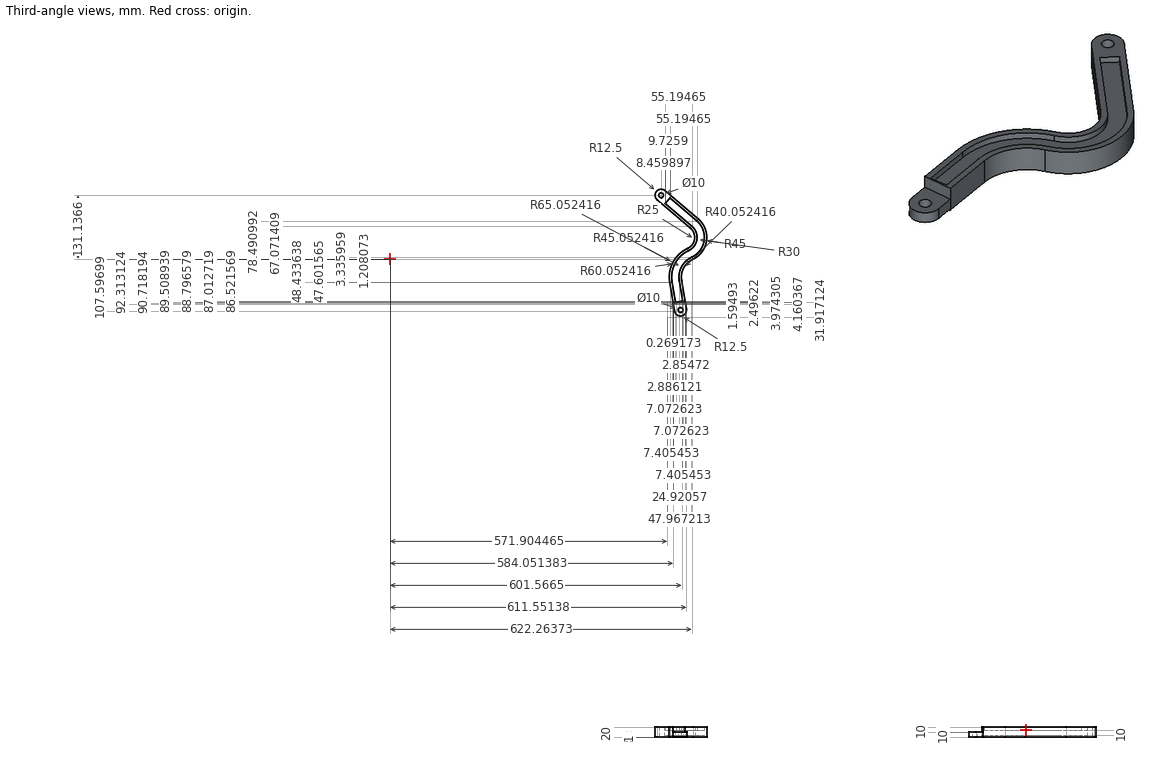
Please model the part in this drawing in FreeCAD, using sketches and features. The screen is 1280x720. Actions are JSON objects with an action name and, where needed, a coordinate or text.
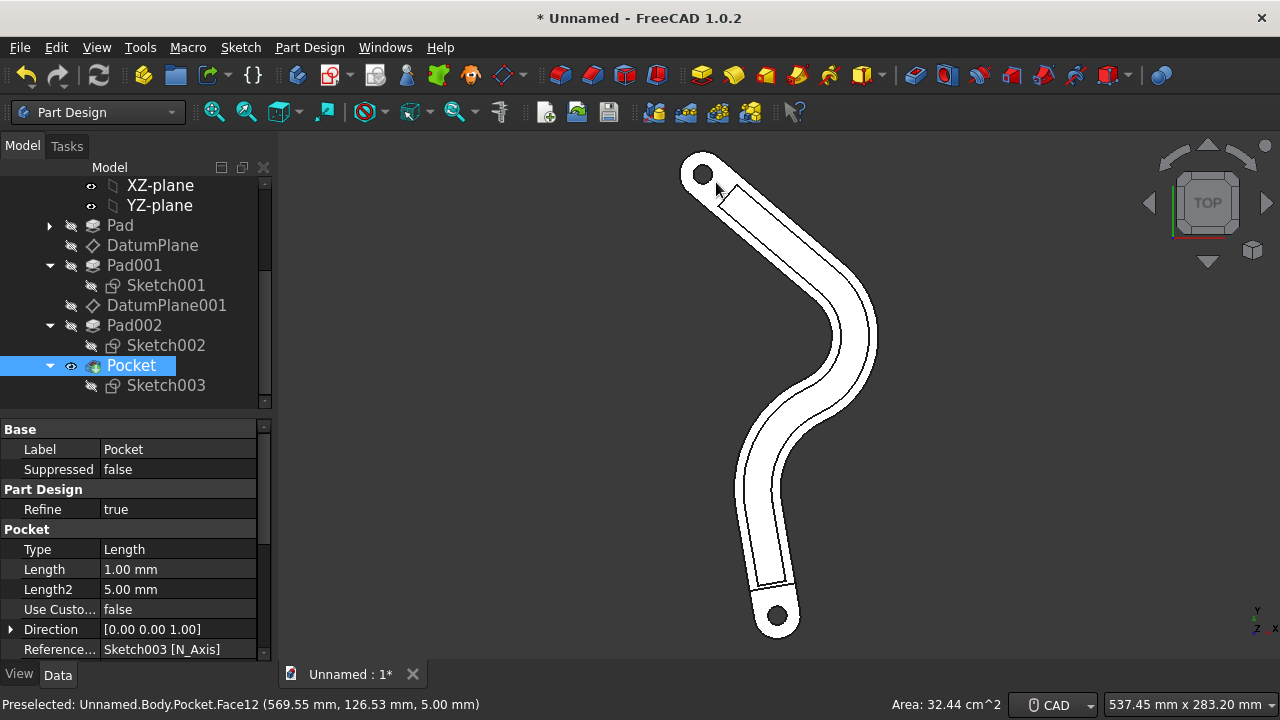
{"action": "left_click", "coordinate": [330, 76]}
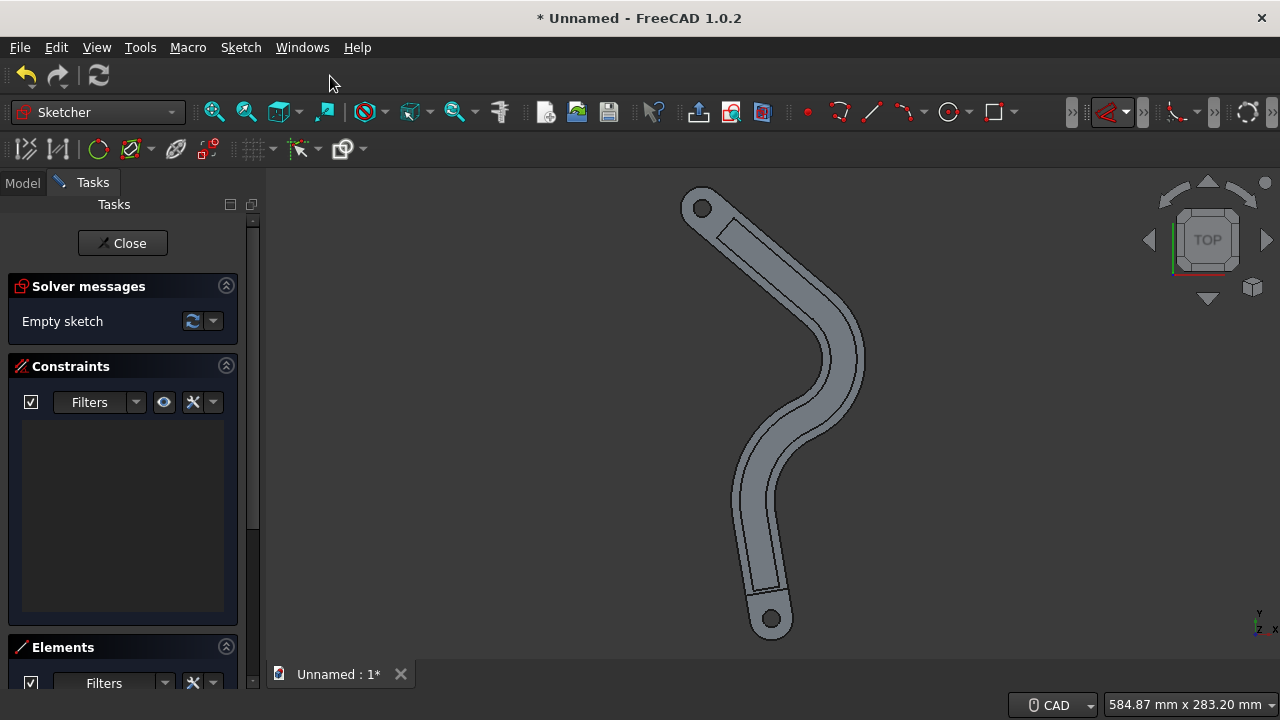
{"action": "scroll", "coordinate": [772, 606], "scroll_direction": "up", "scroll_amount": 13}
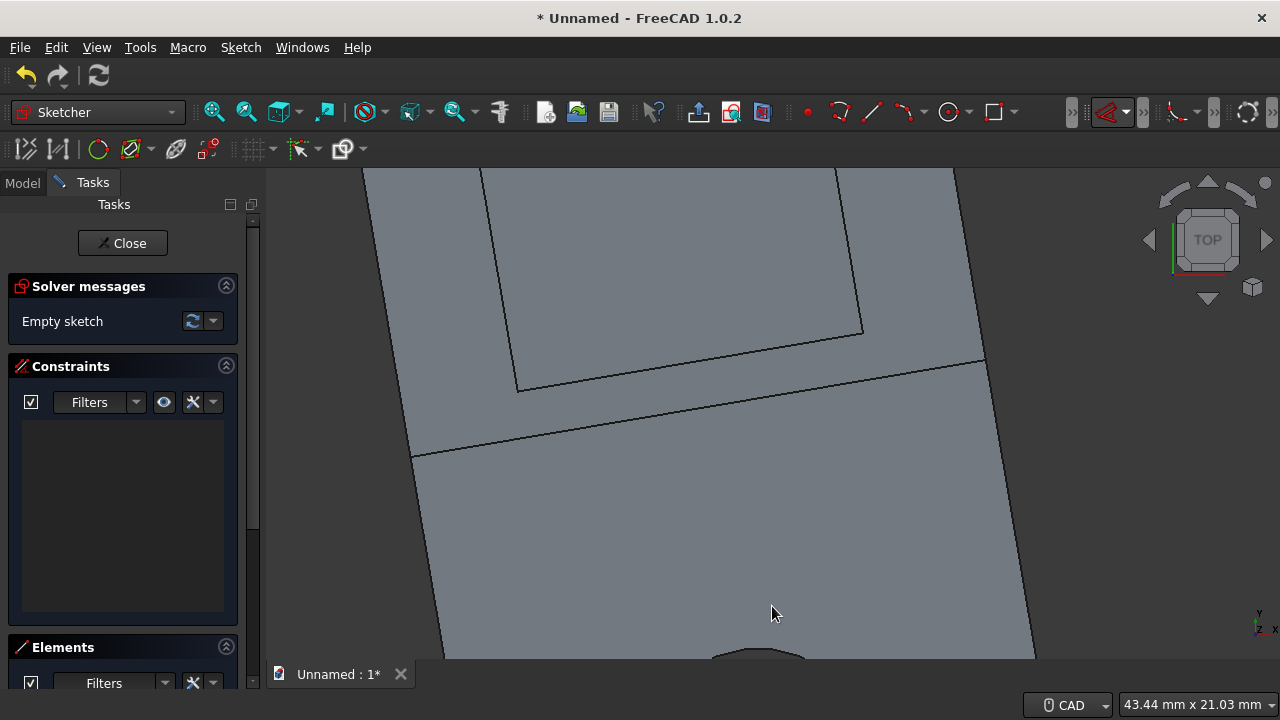
{"action": "left_click", "coordinate": [840, 112]}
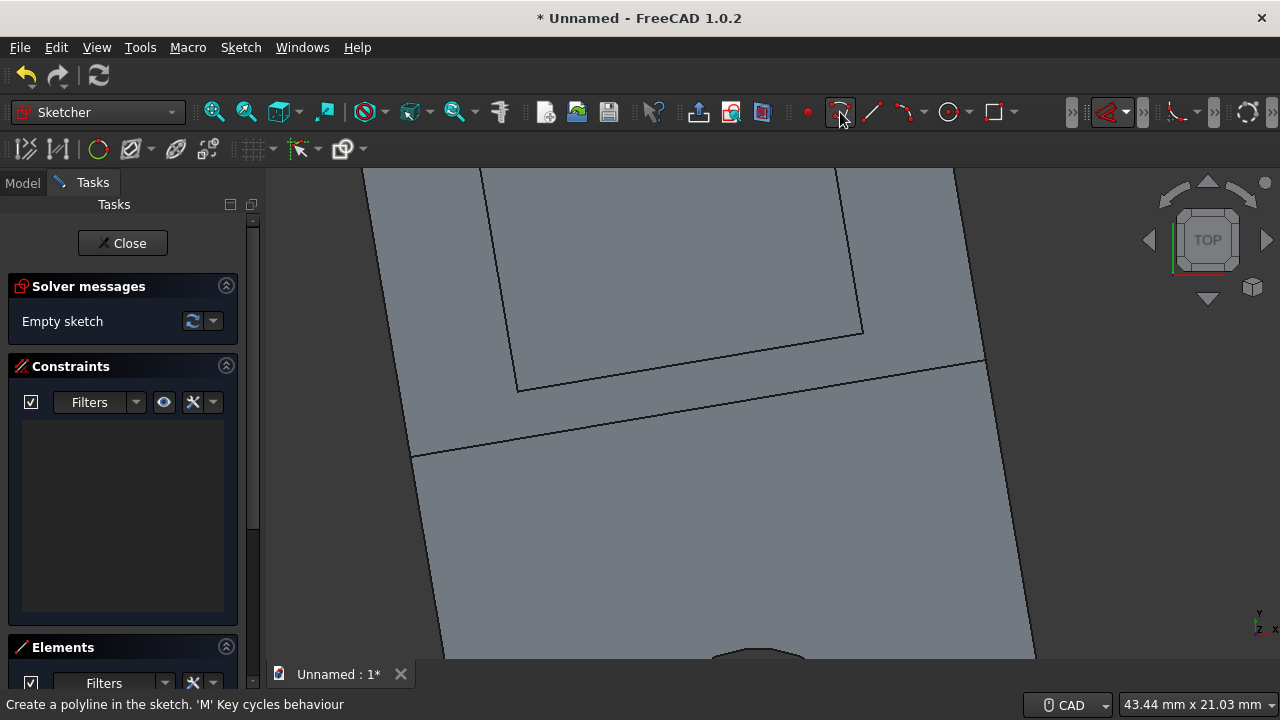
{"action": "left_click", "coordinate": [404, 420]}
{"action": "left_click", "coordinate": [410, 457]}
{"action": "left_click", "coordinate": [986, 360]}
{"action": "left_click", "coordinate": [404, 421]}
{"action": "key", "text": "Escape"}
{"action": "key", "text": "Escape"}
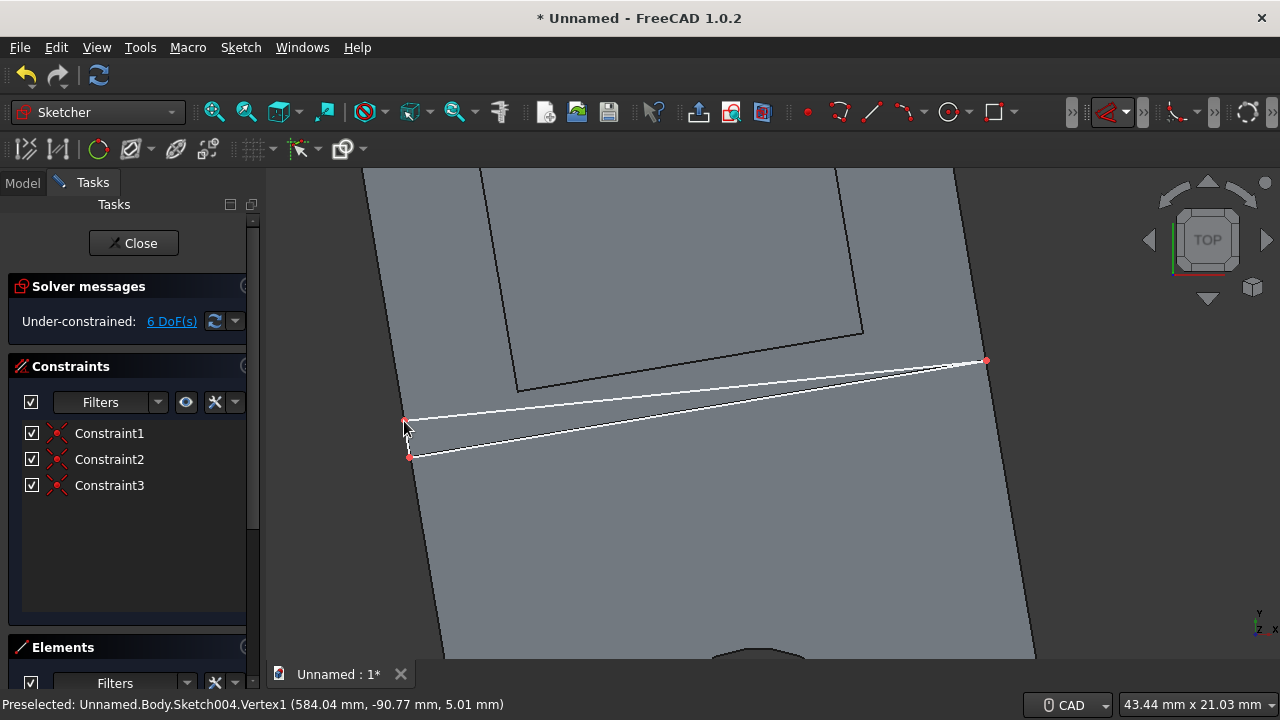
{"action": "scroll", "coordinate": [406, 432], "scroll_direction": "up", "scroll_amount": 2}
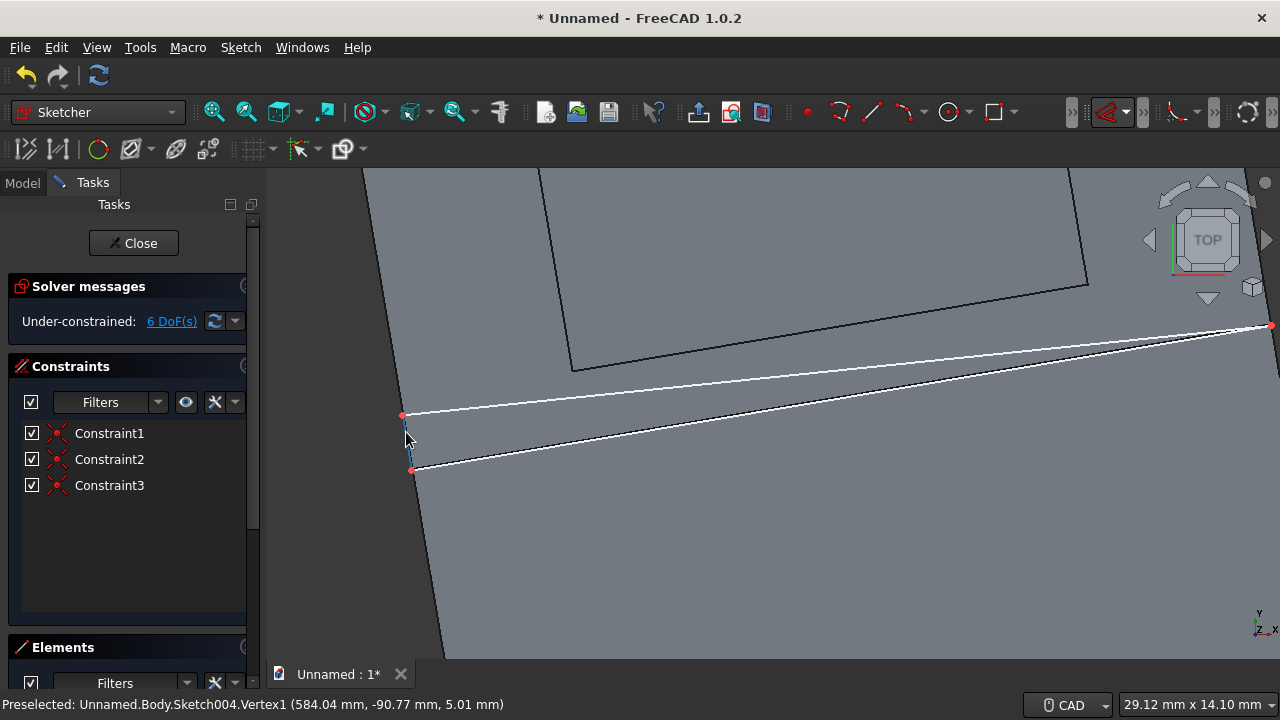
{"action": "left_click", "coordinate": [406, 432]}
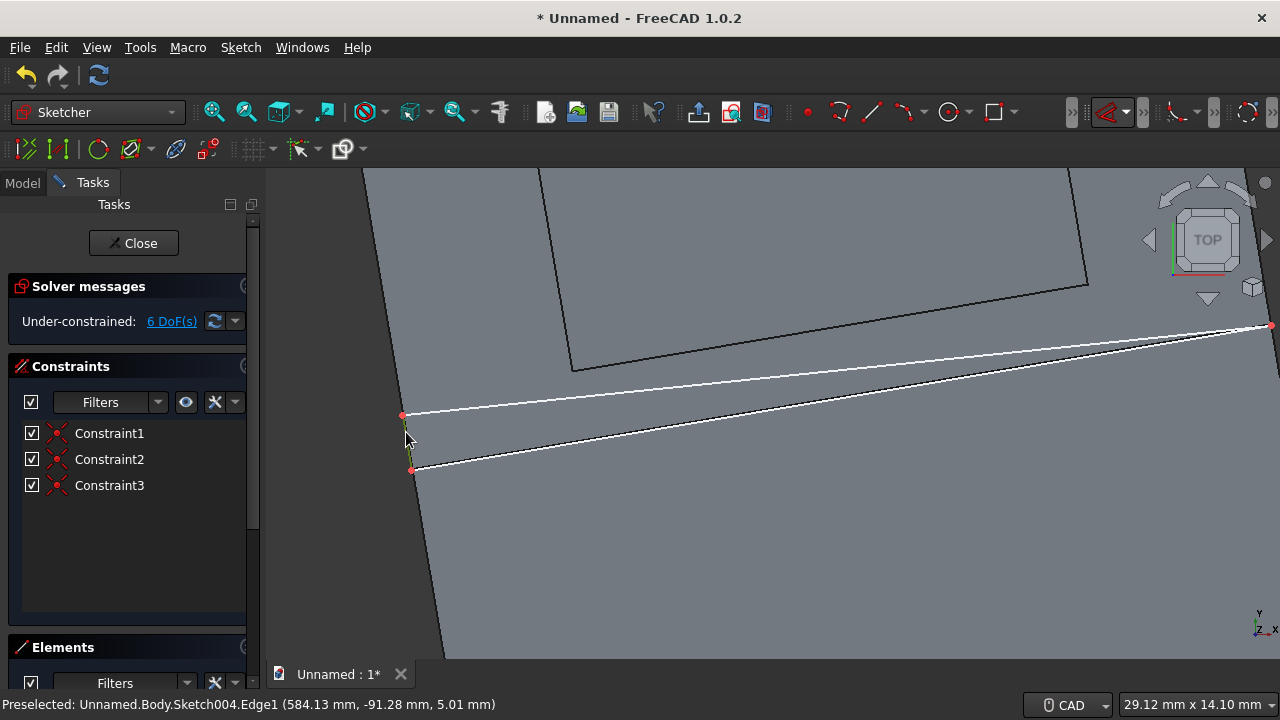
{"action": "left_click", "coordinate": [1128, 112]}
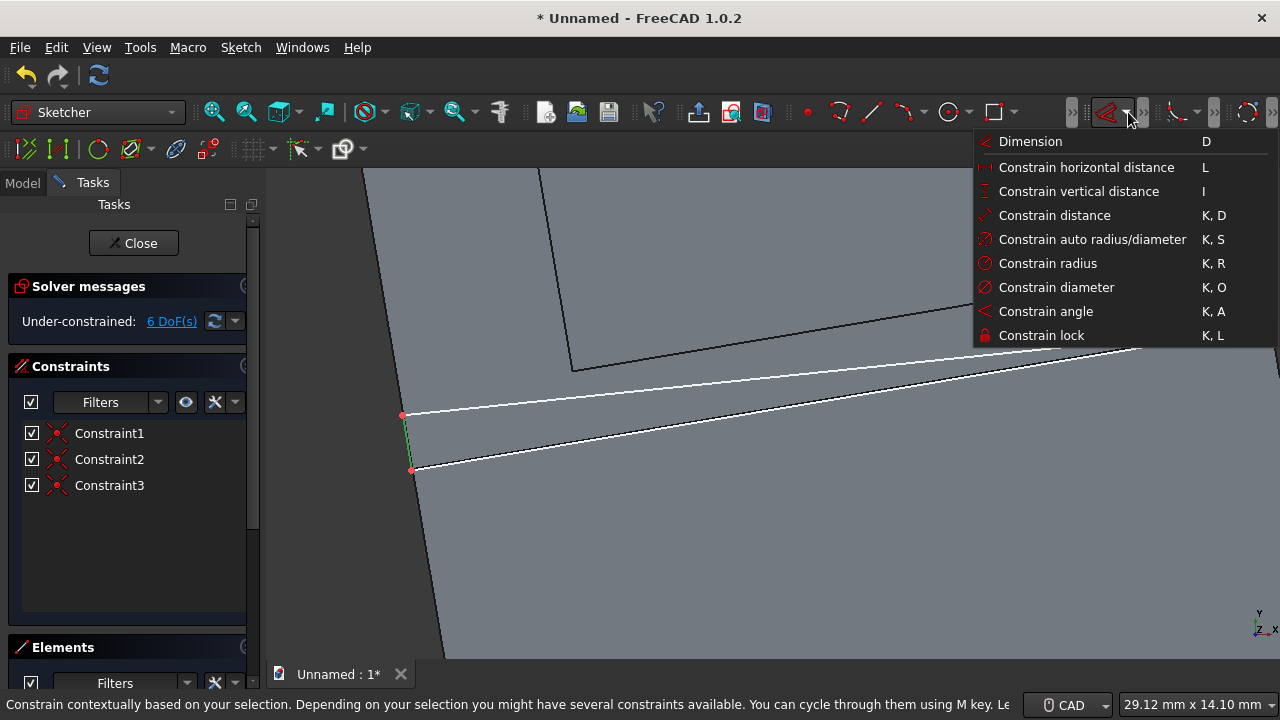
{"action": "left_click", "coordinate": [1126, 191]}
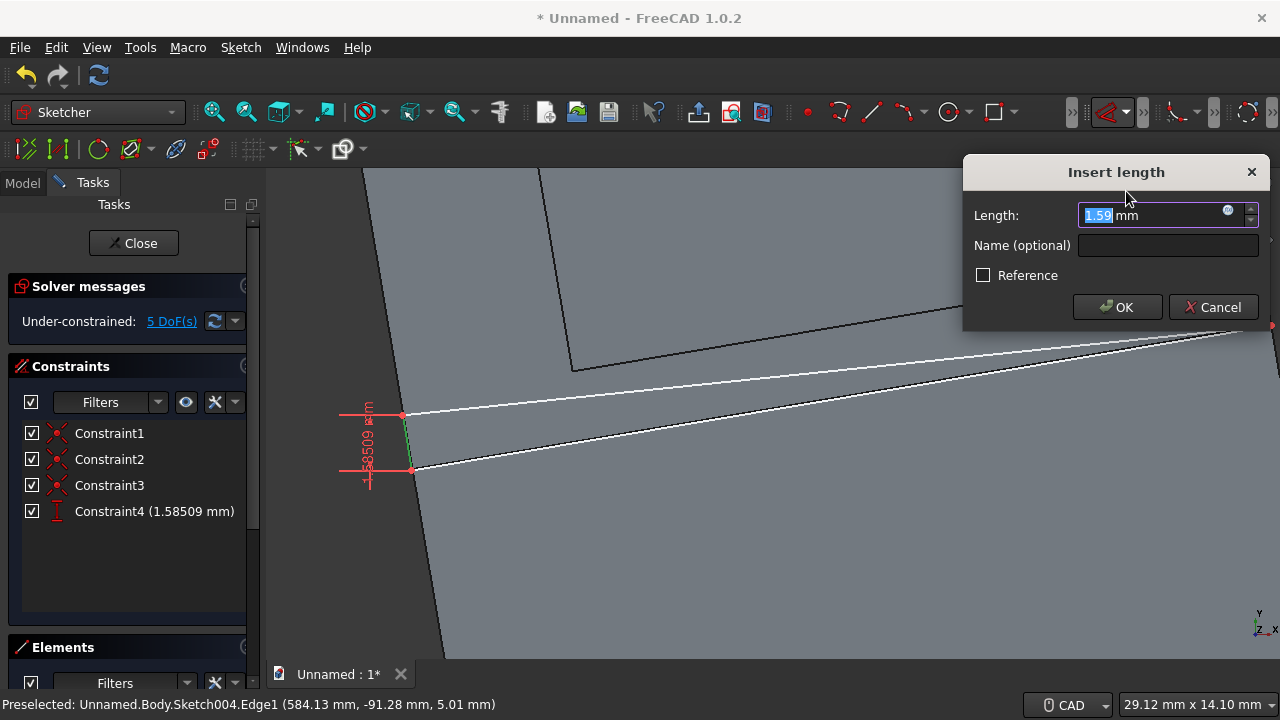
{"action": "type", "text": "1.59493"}
{"action": "key", "text": "Return"}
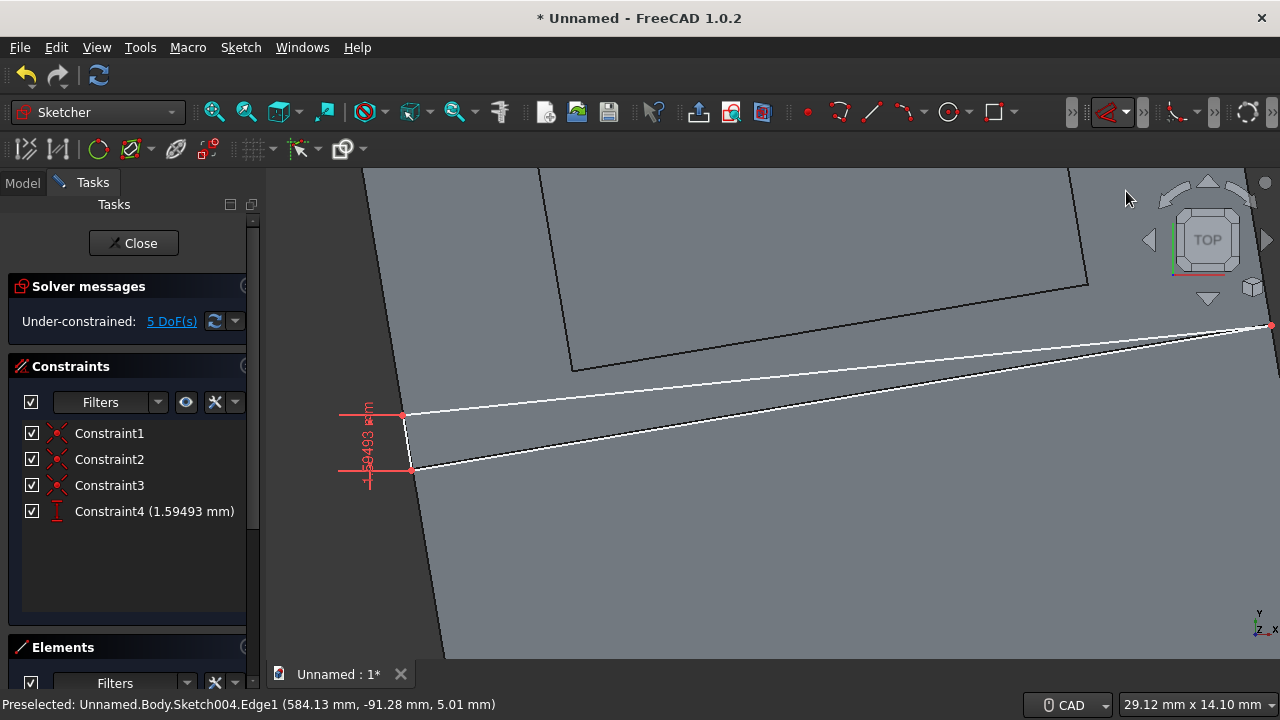
{"action": "scroll", "coordinate": [406, 432], "scroll_direction": "up", "scroll_amount": 8}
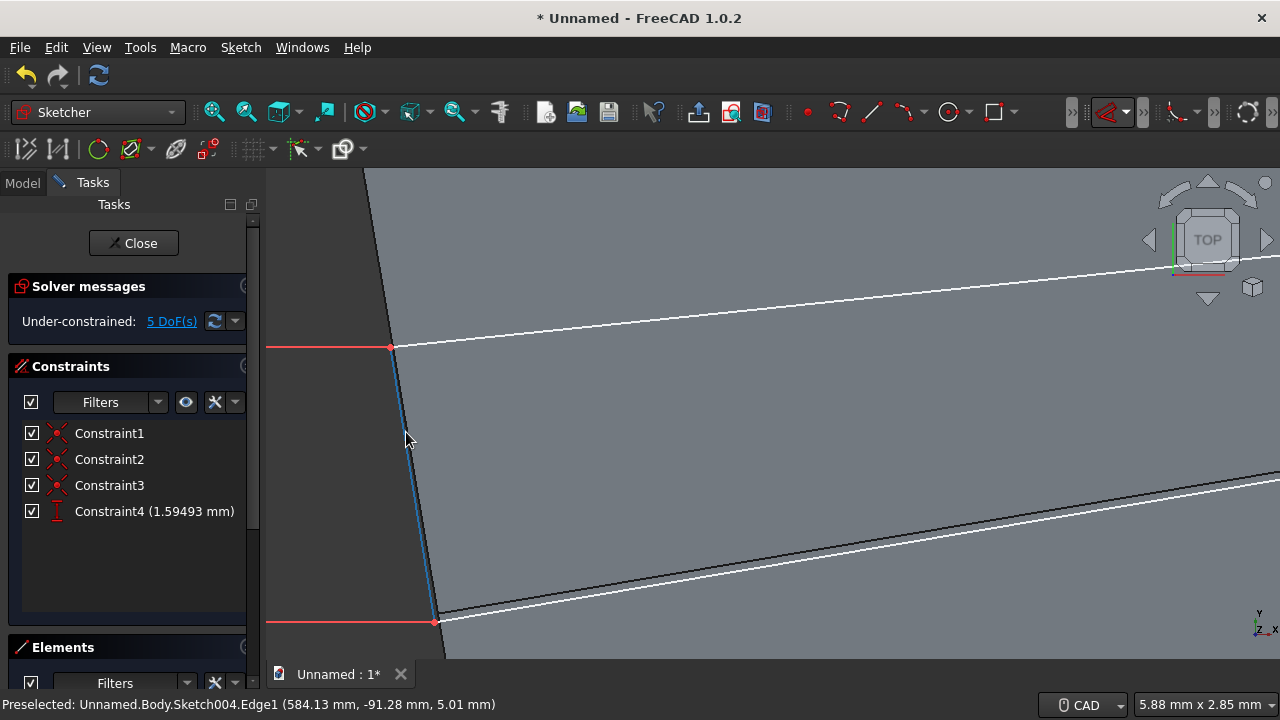
{"action": "left_click", "coordinate": [404, 430]}